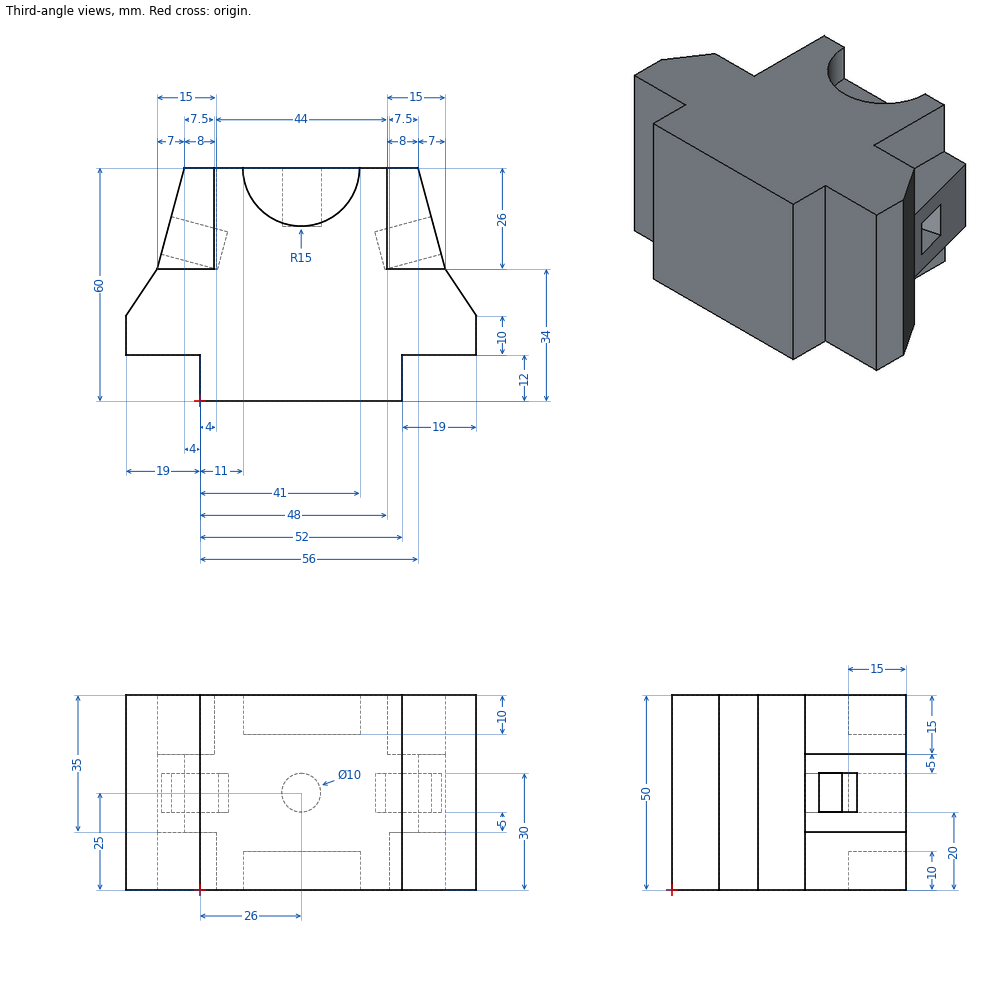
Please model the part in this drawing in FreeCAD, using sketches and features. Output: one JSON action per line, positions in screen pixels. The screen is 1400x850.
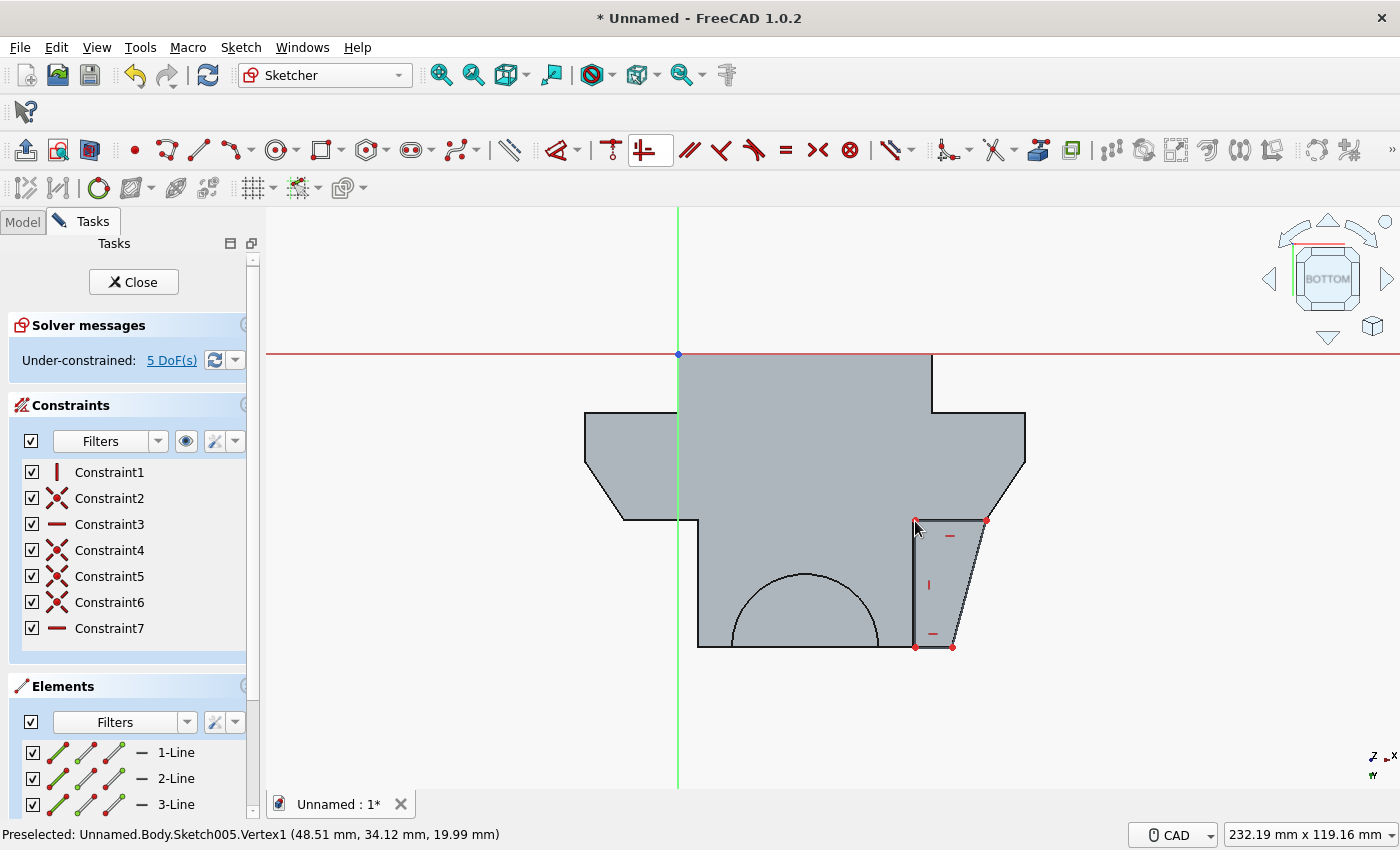
{"action": "left_click", "coordinate": [556, 150]}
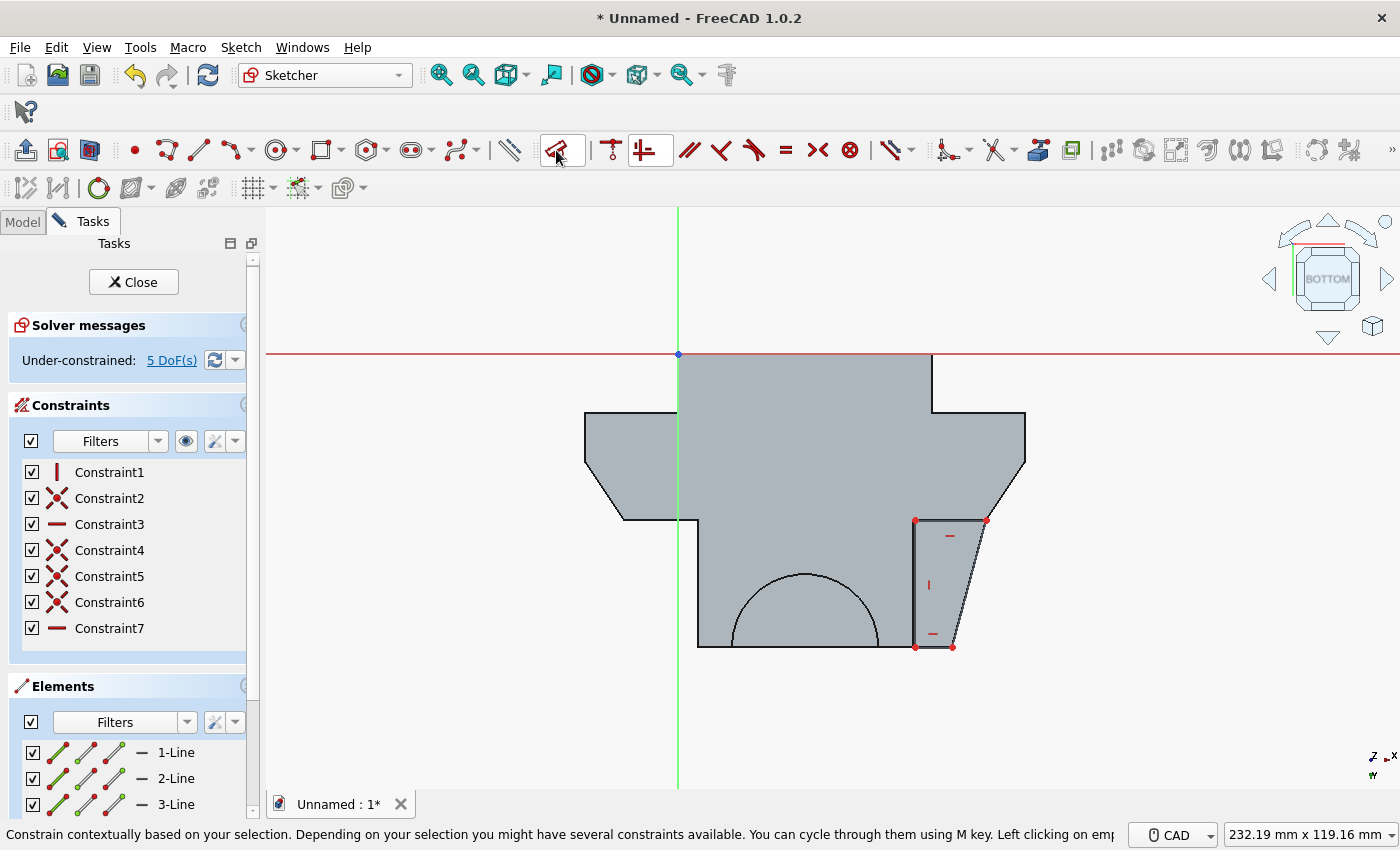
{"action": "left_click", "coordinate": [915, 559]}
{"action": "left_click", "coordinate": [949, 585]}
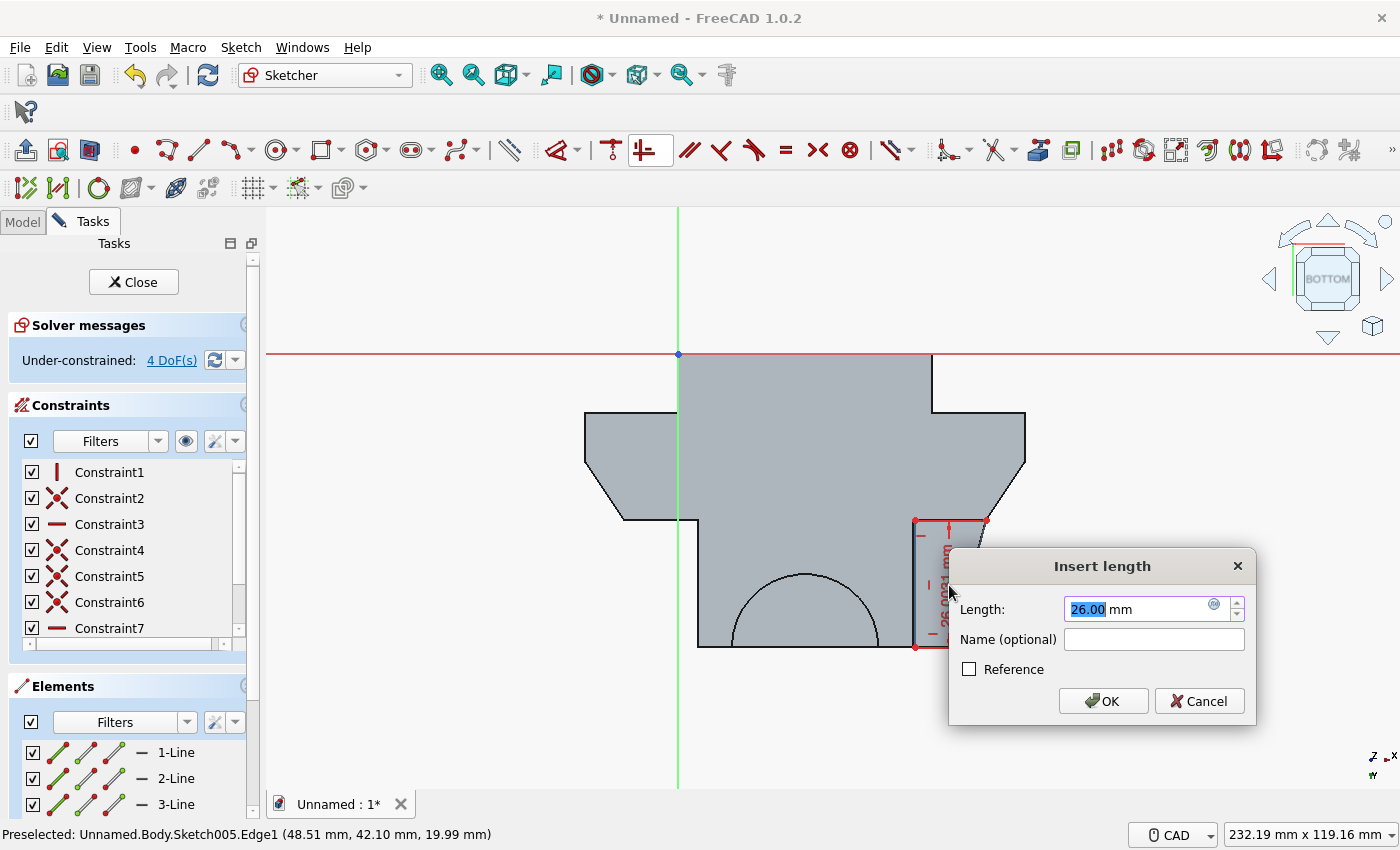
{"action": "type", "text": "26"}
{"action": "key", "text": "Return"}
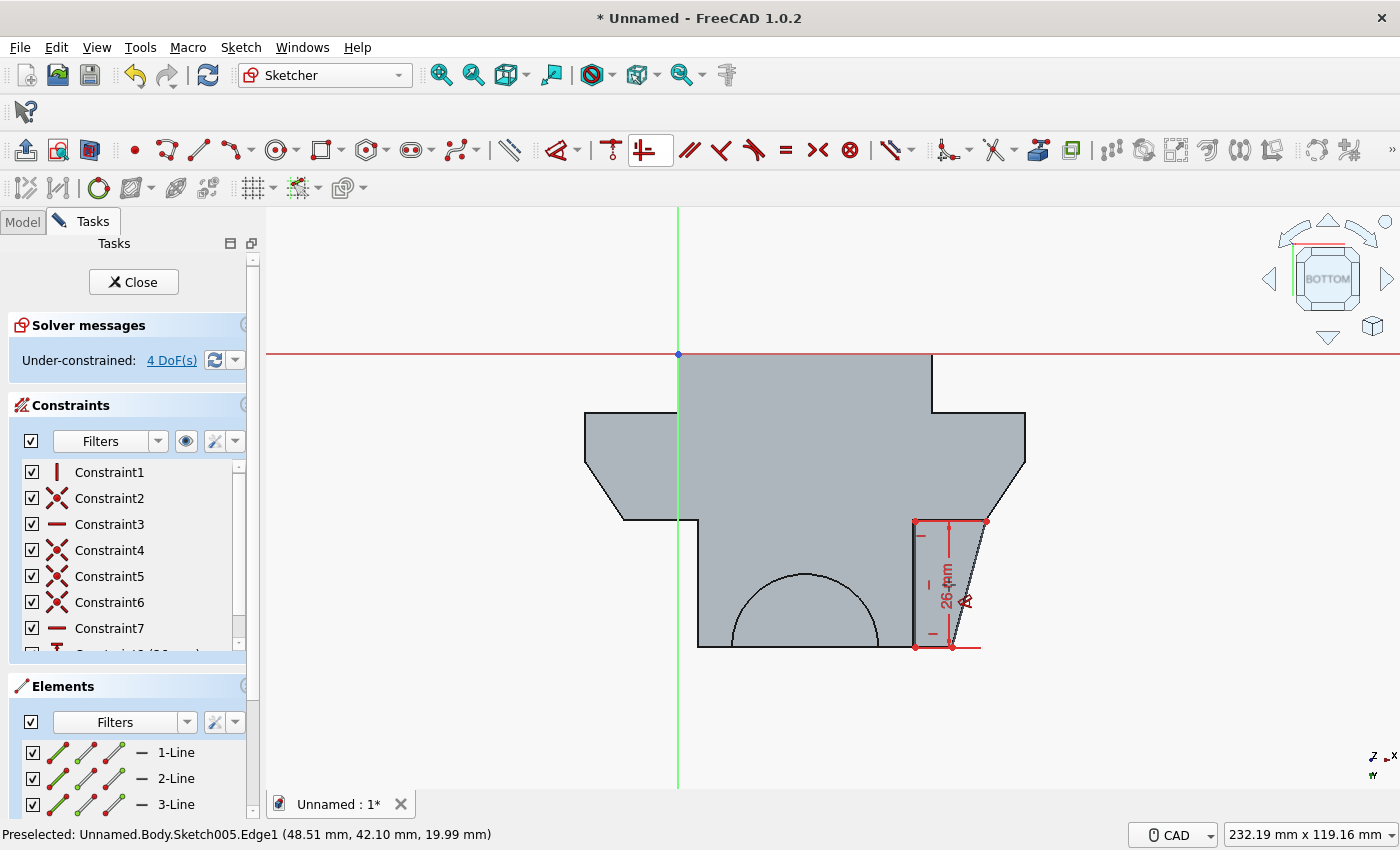
{"action": "left_click", "coordinate": [962, 610]}
{"action": "left_click", "coordinate": [969, 682]}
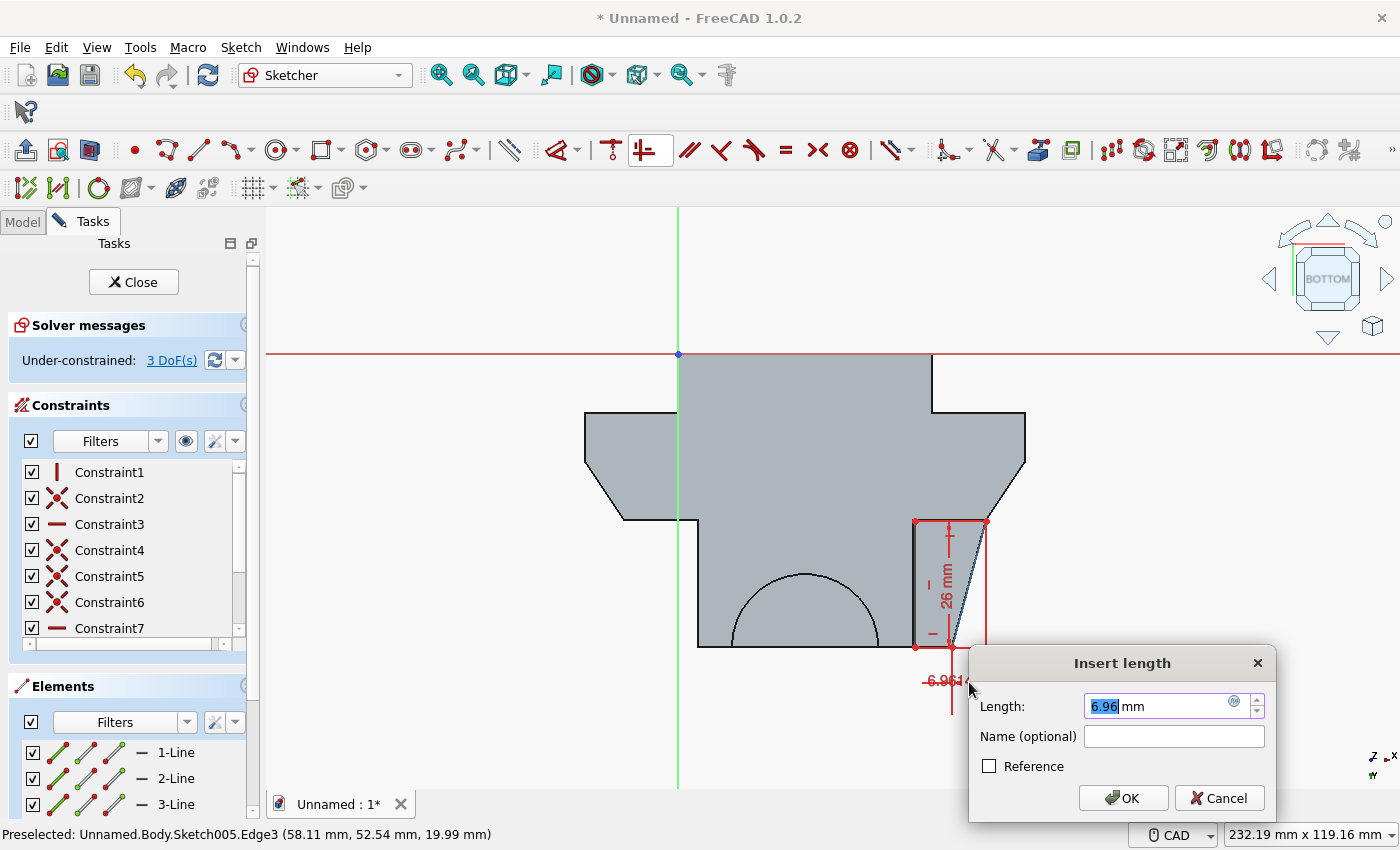
{"action": "type", "text": "7"}
{"action": "key", "text": "Return"}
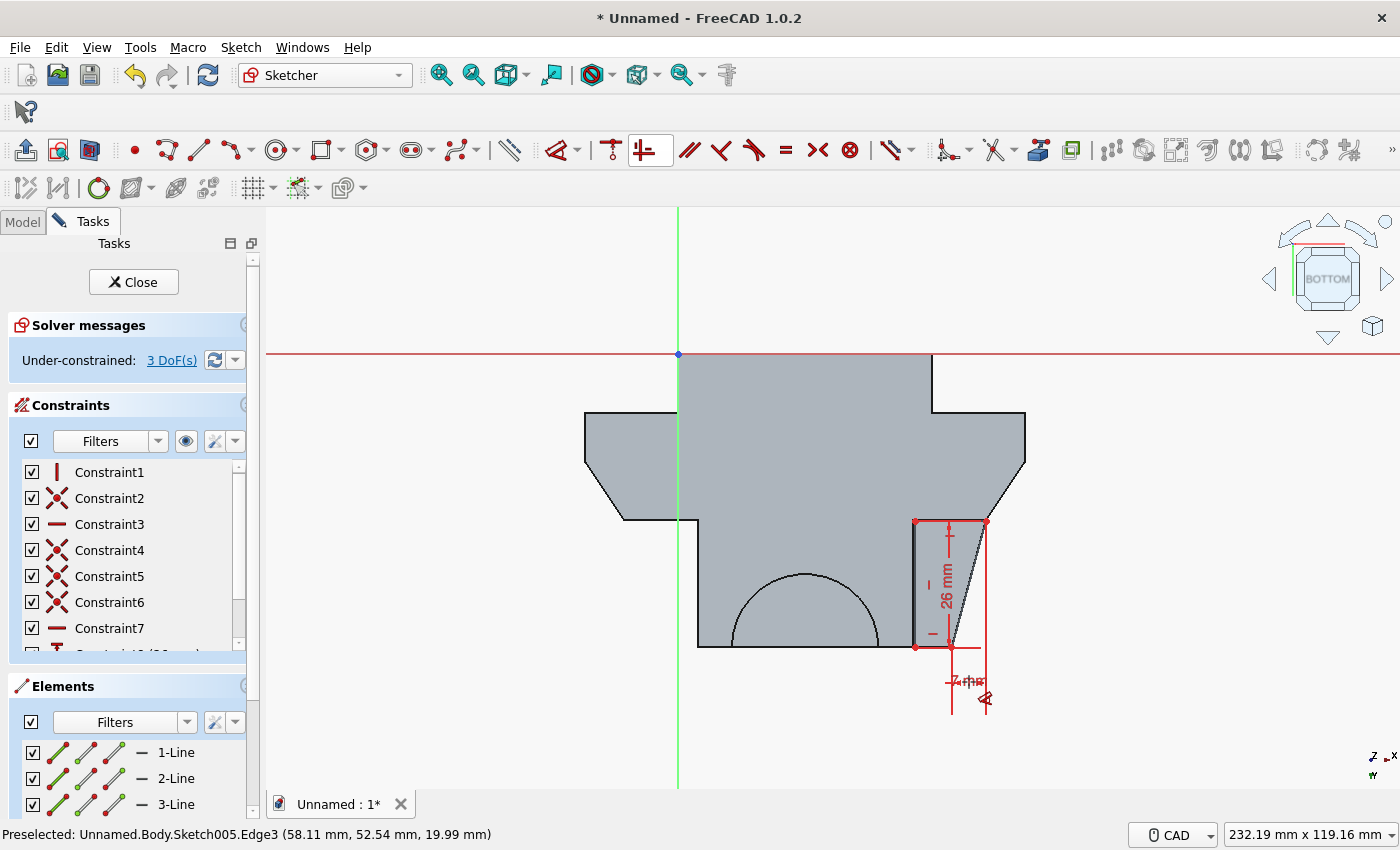
{"action": "scroll", "coordinate": [926, 648], "scroll_direction": "up", "scroll_amount": 2}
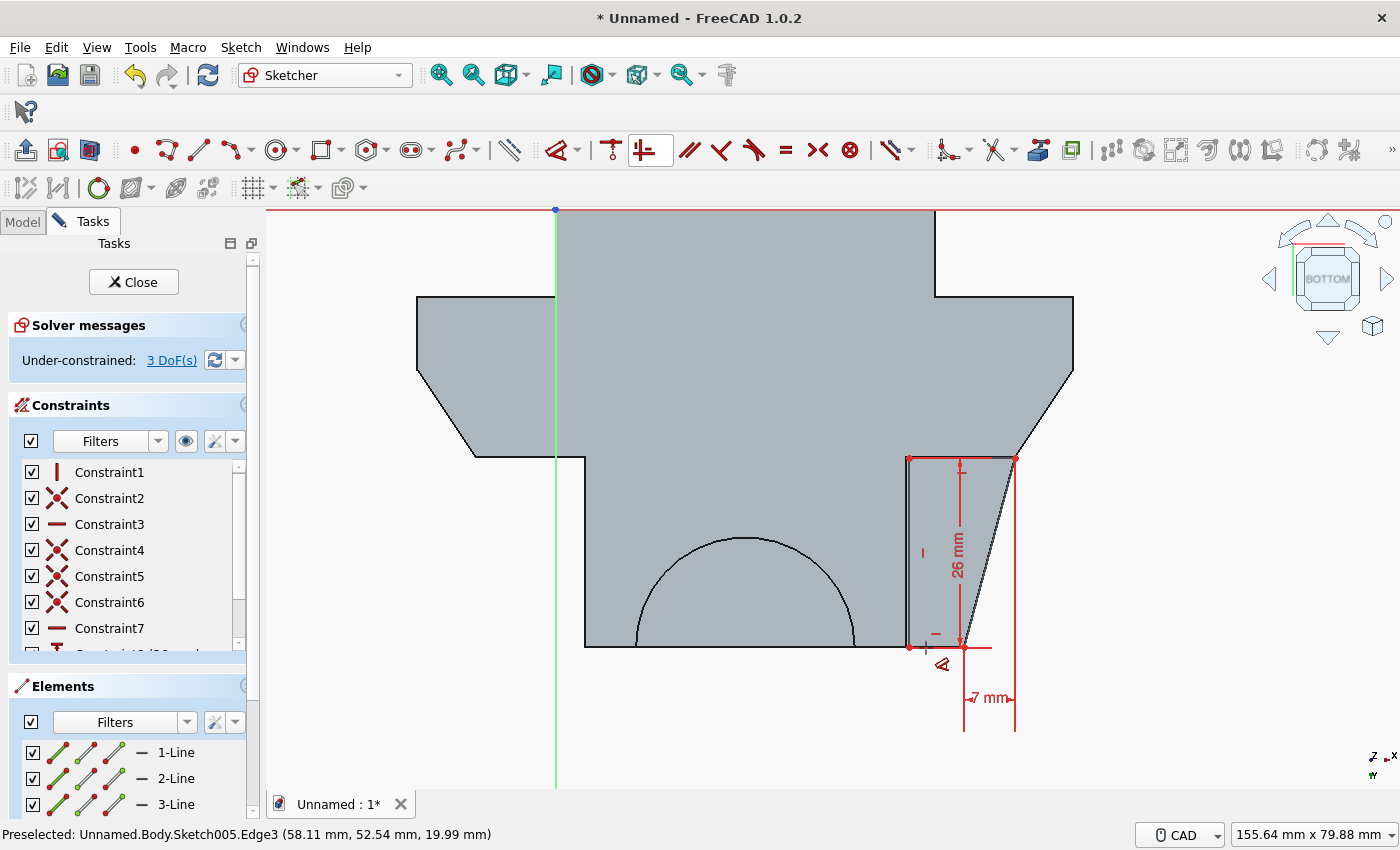
{"action": "left_click", "coordinate": [926, 648]}
{"action": "left_click", "coordinate": [918, 682]}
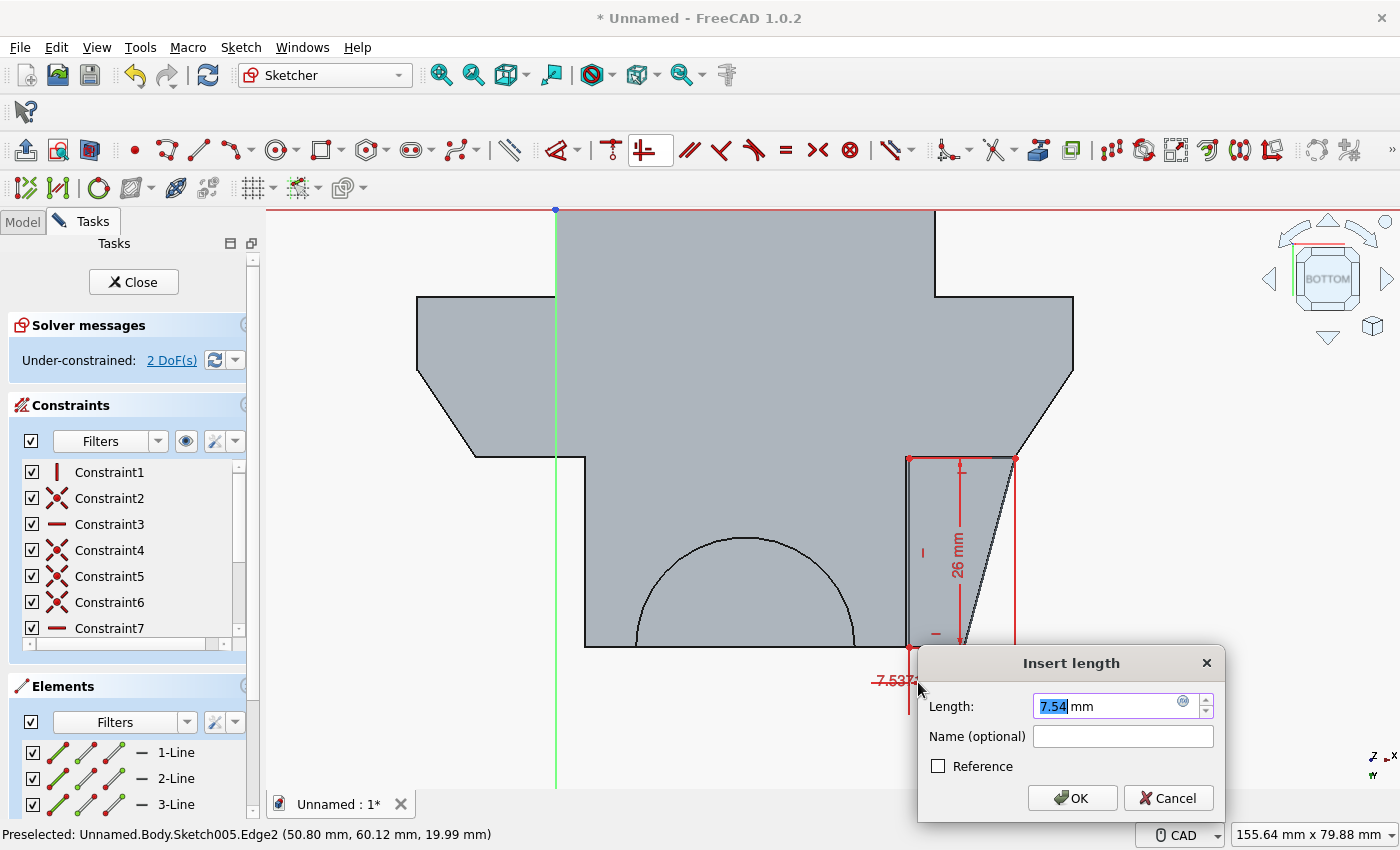
{"action": "type", "text": "7.5"}
{"action": "key", "text": "Return"}